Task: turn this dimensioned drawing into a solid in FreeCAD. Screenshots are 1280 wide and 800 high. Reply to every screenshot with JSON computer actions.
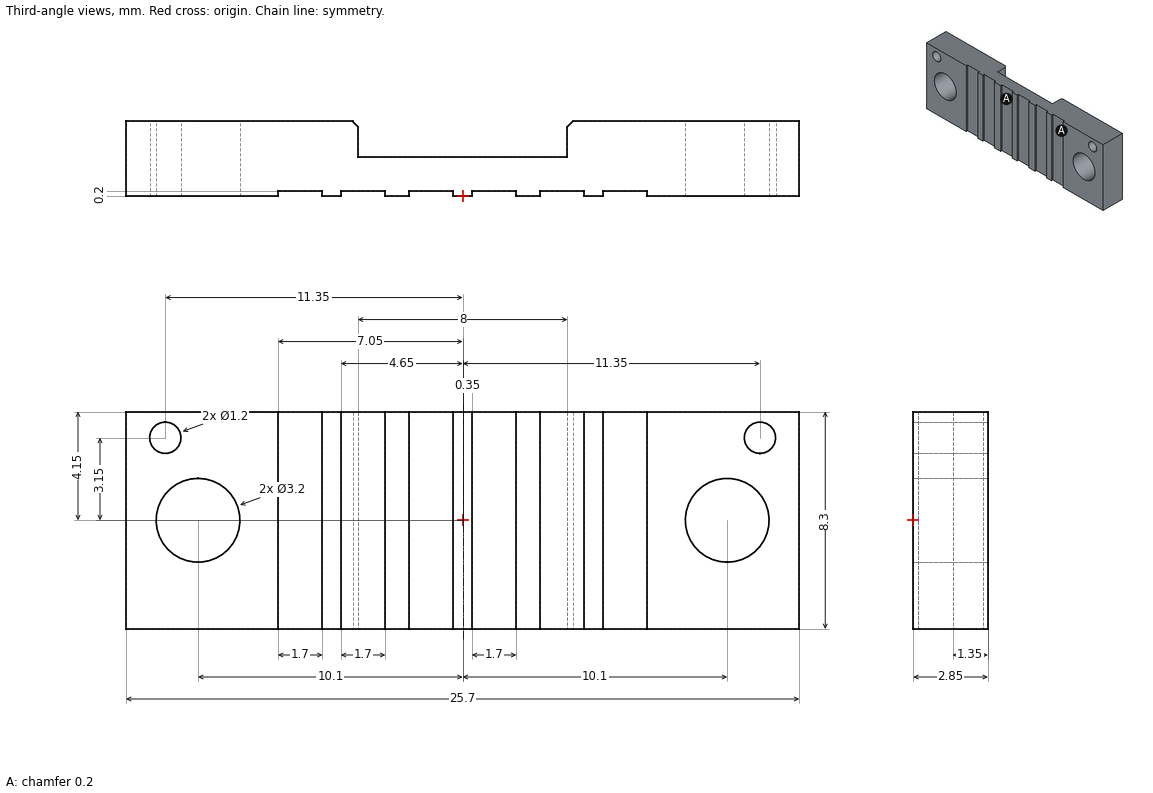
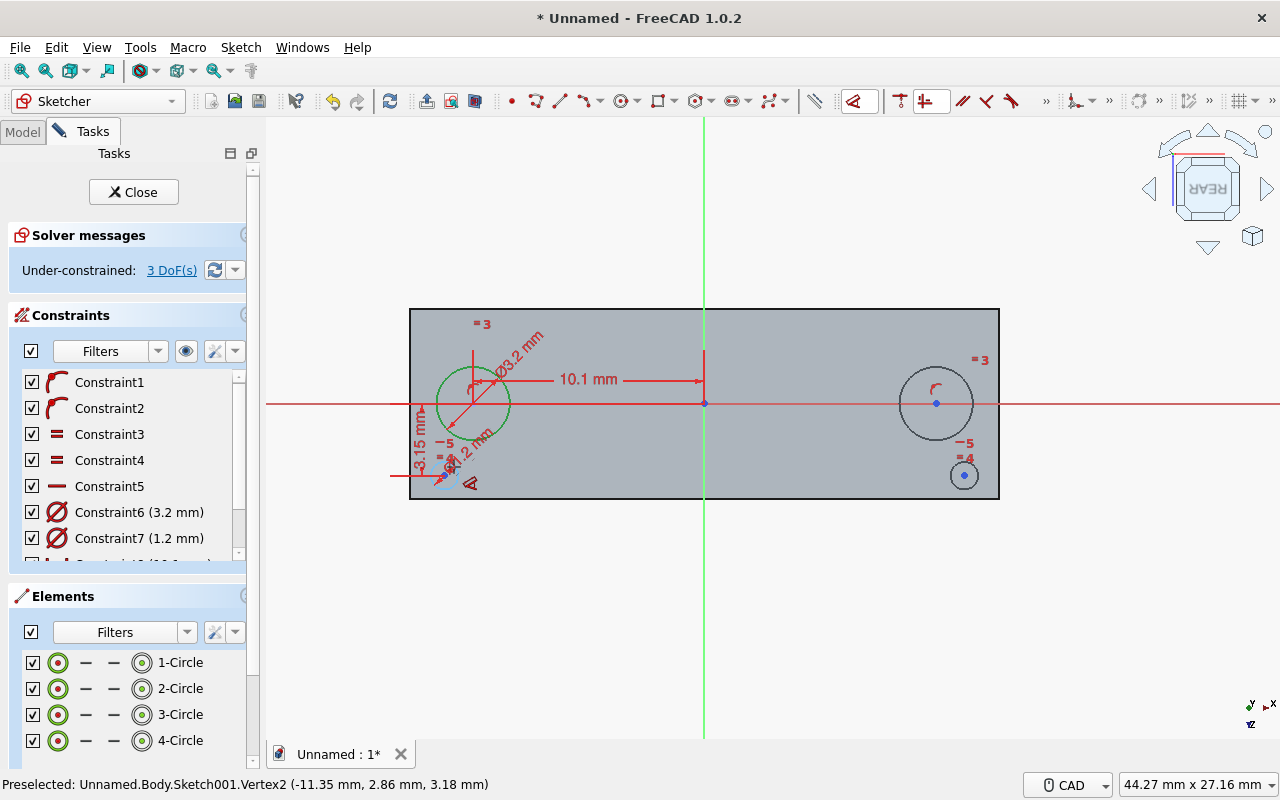
{"action": "left_click", "coordinate": [936, 404]}
{"action": "left_click", "coordinate": [820, 370]}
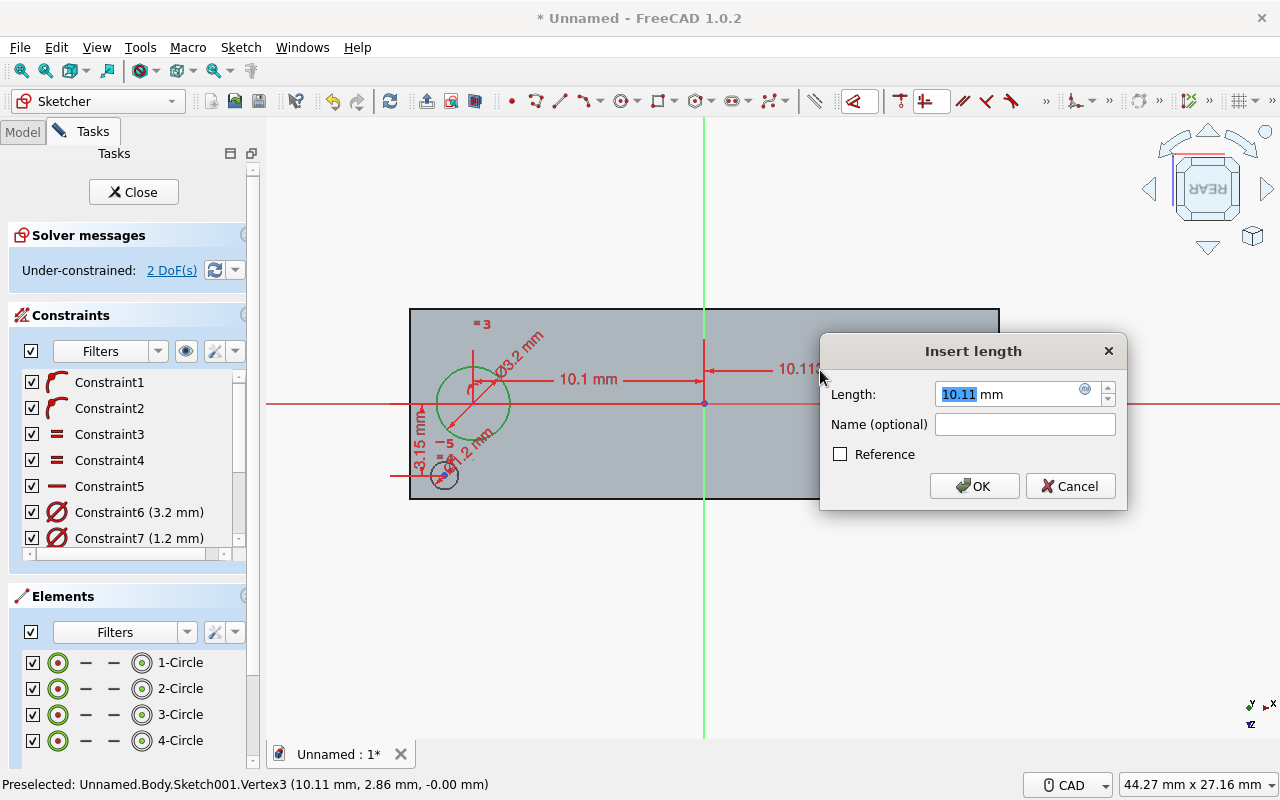
{"action": "type", "text": "10.1"}
{"action": "key", "text": "Return"}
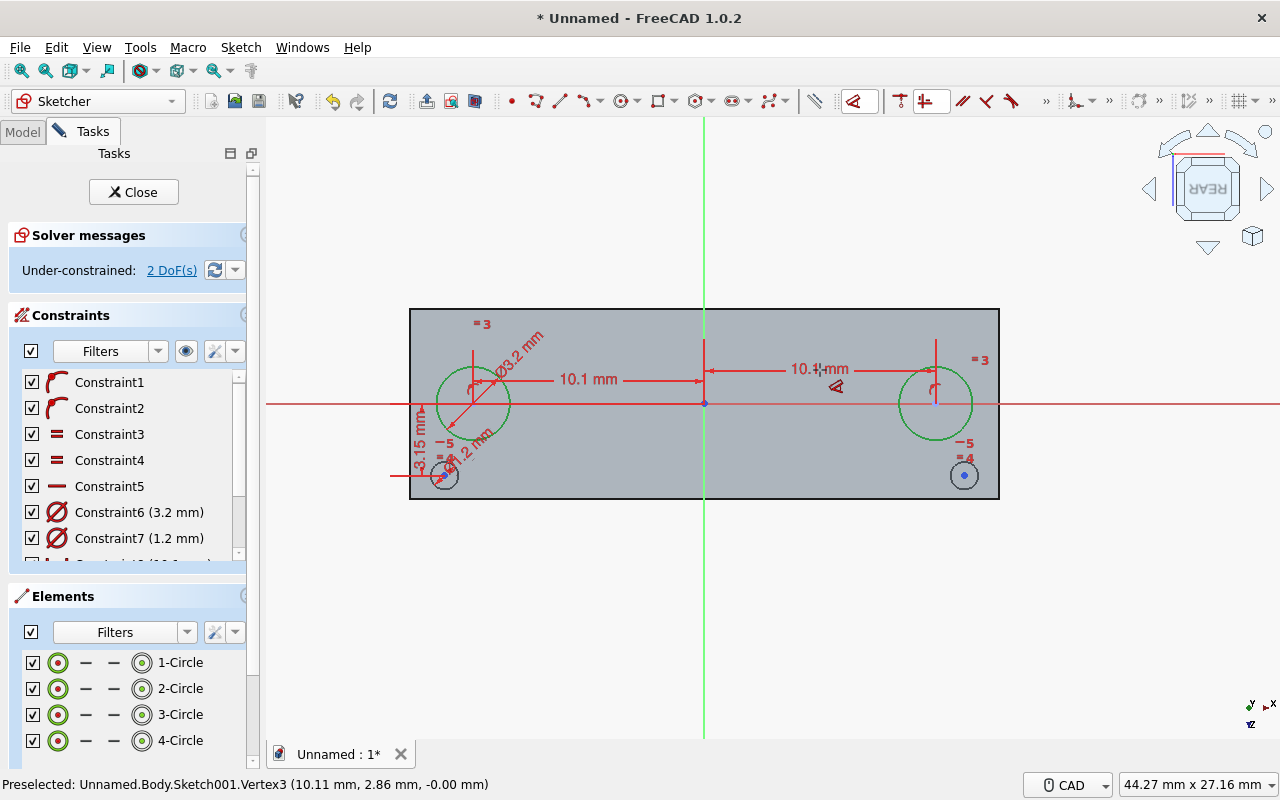
{"action": "left_click", "coordinate": [445, 476]}
{"action": "left_click", "coordinate": [575, 510]}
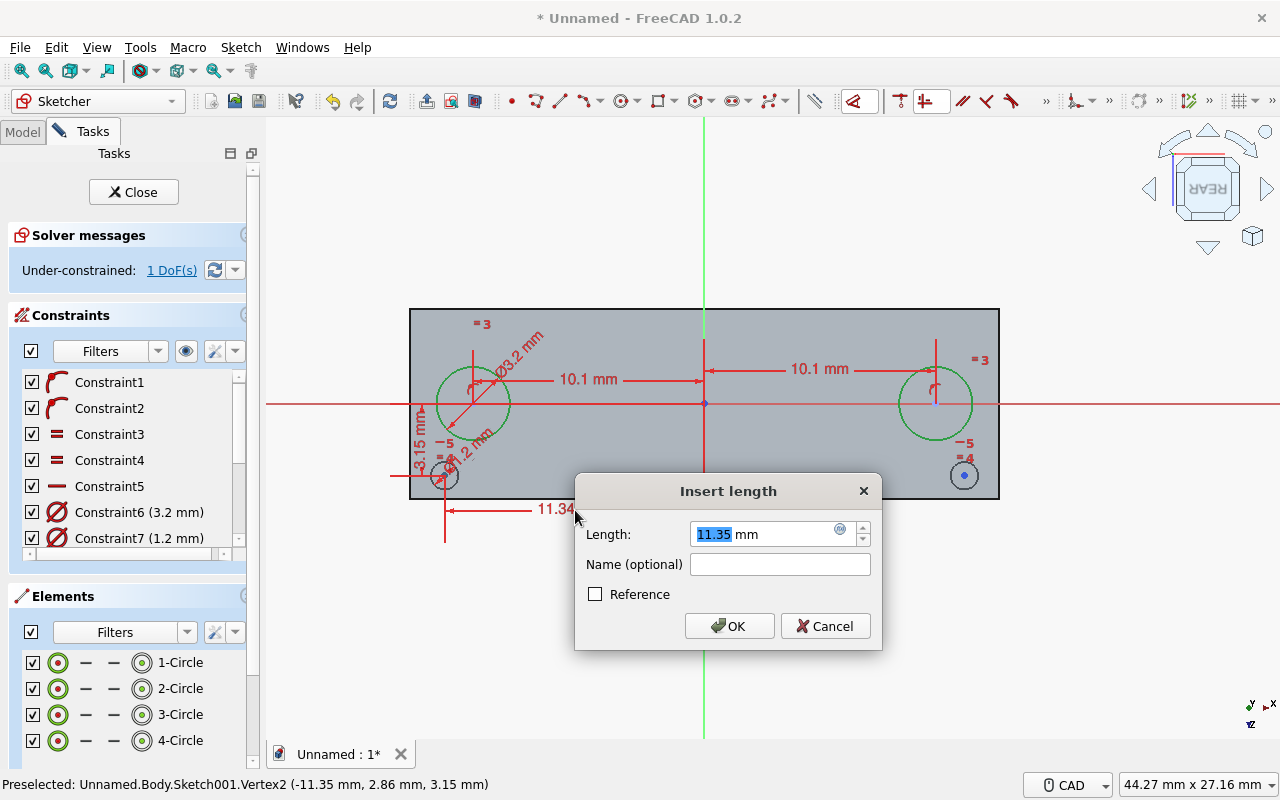
{"action": "type", "text": "11.35"}
{"action": "key", "text": "Return"}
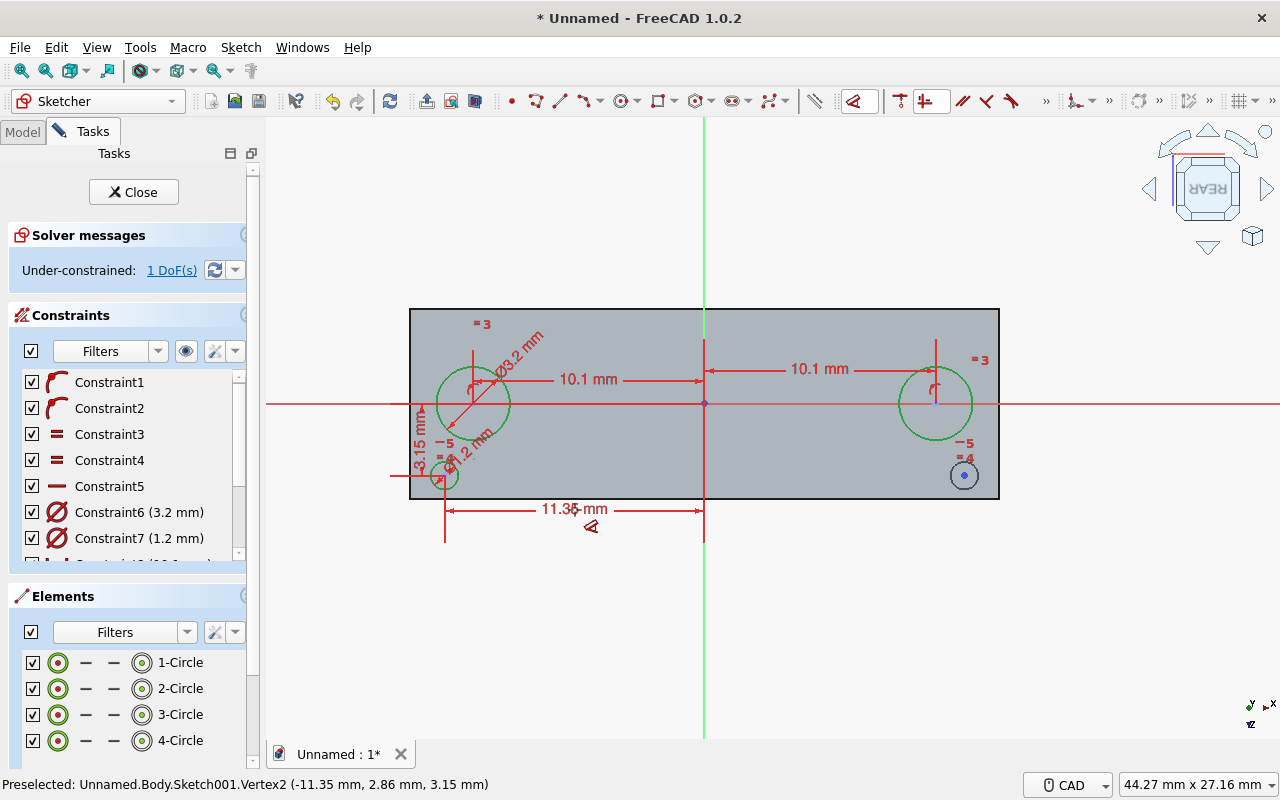
{"action": "left_click", "coordinate": [964, 476]}
{"action": "left_click", "coordinate": [834, 510]}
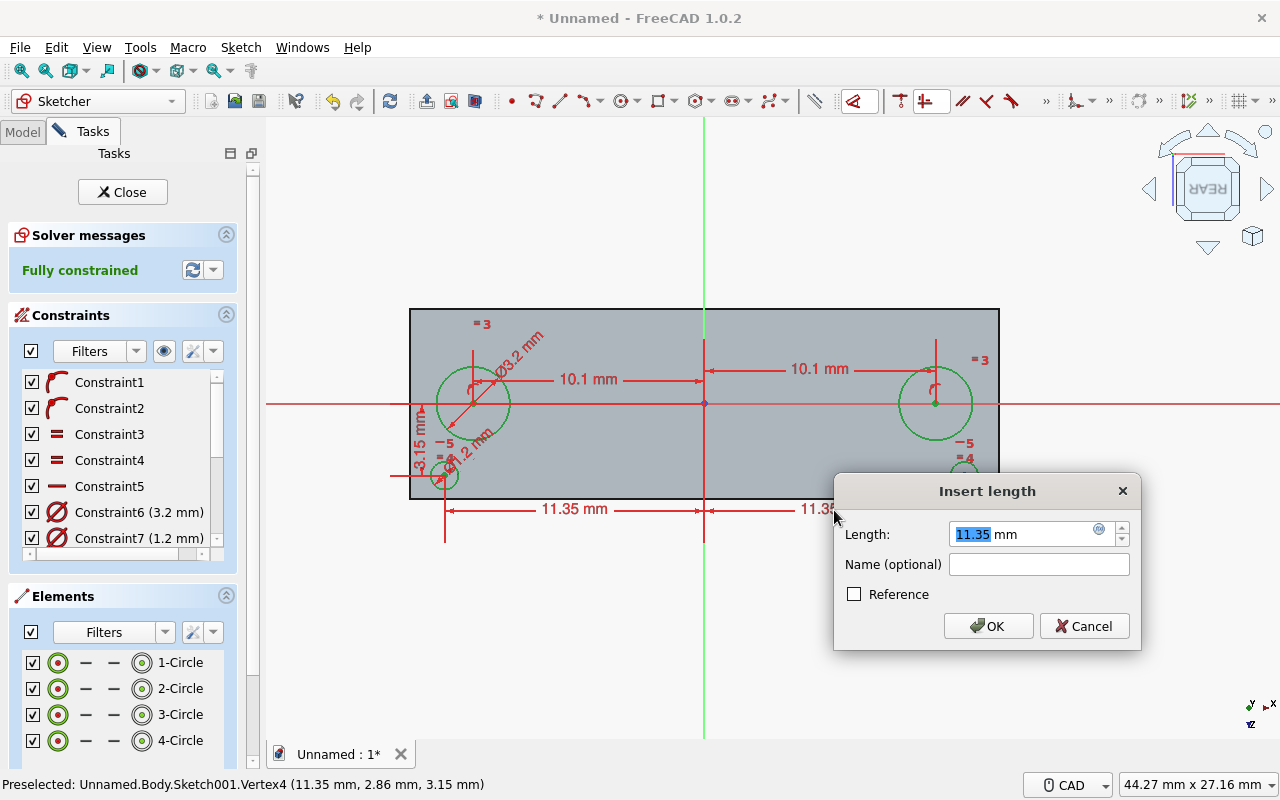
{"action": "type", "text": "11.35"}
{"action": "key", "text": "Return"}
{"action": "key", "text": "Escape"}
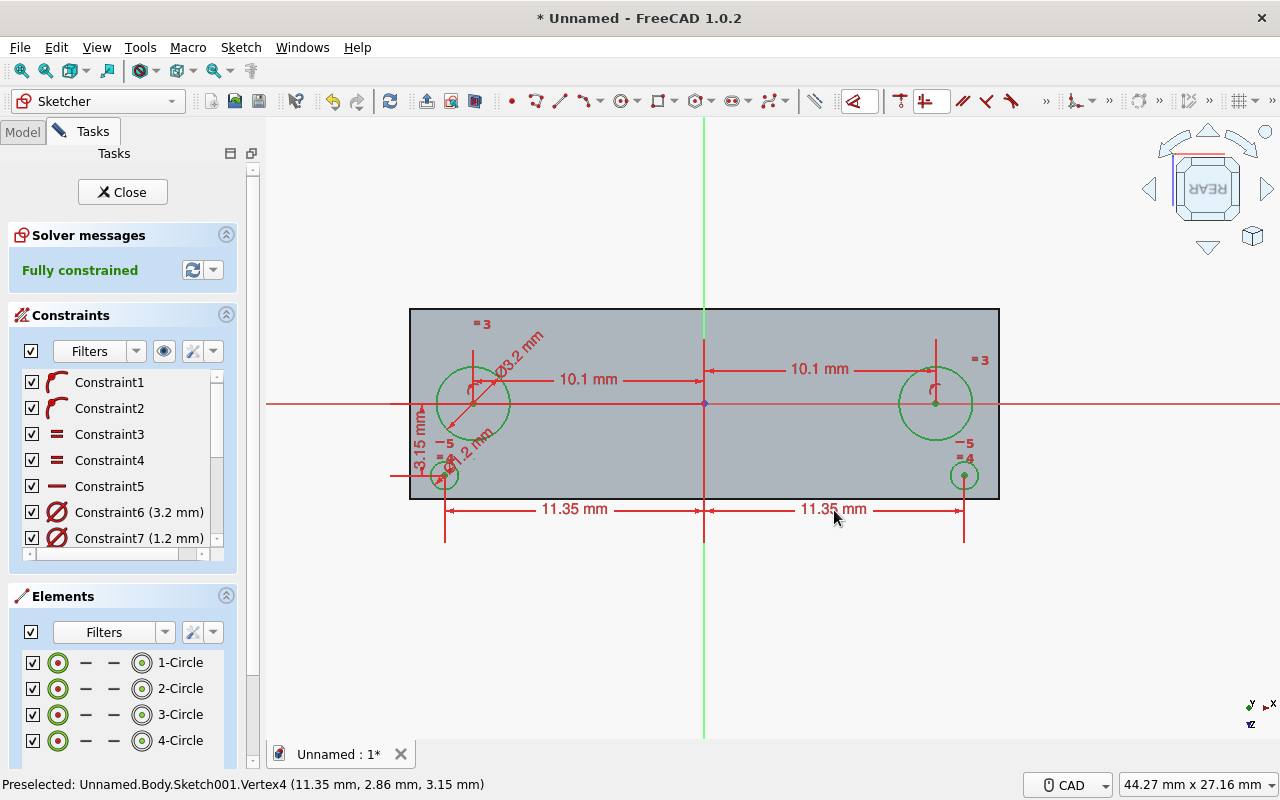
{"action": "left_click", "coordinate": [123, 192]}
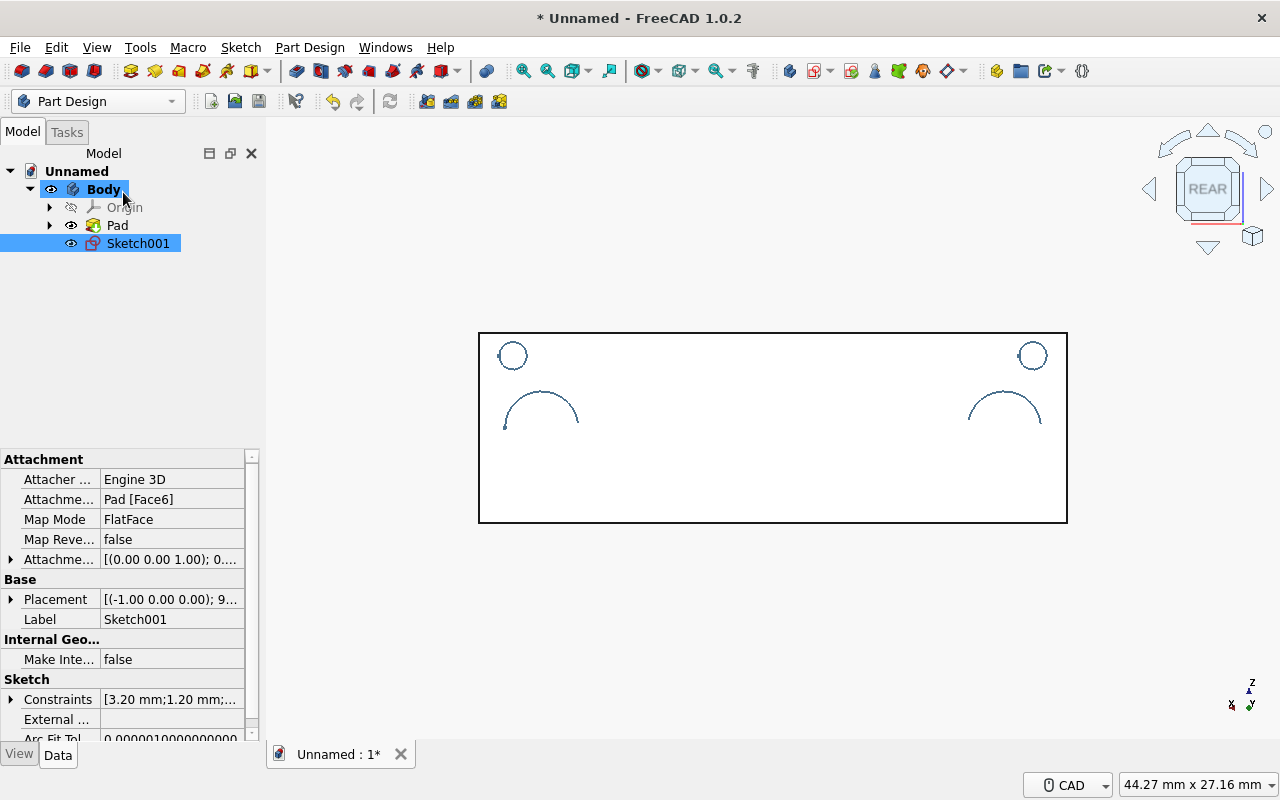
{"action": "left_click", "coordinate": [298, 72]}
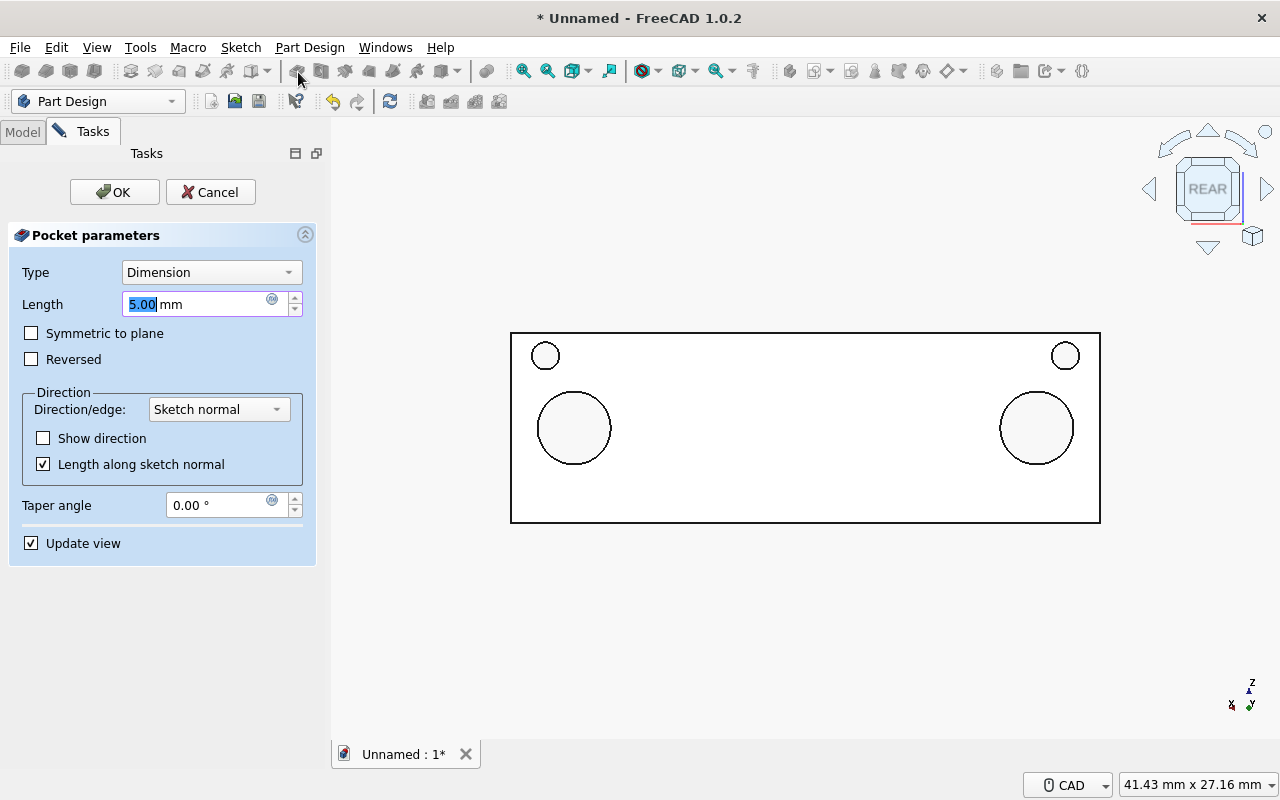
{"action": "left_click", "coordinate": [212, 272]}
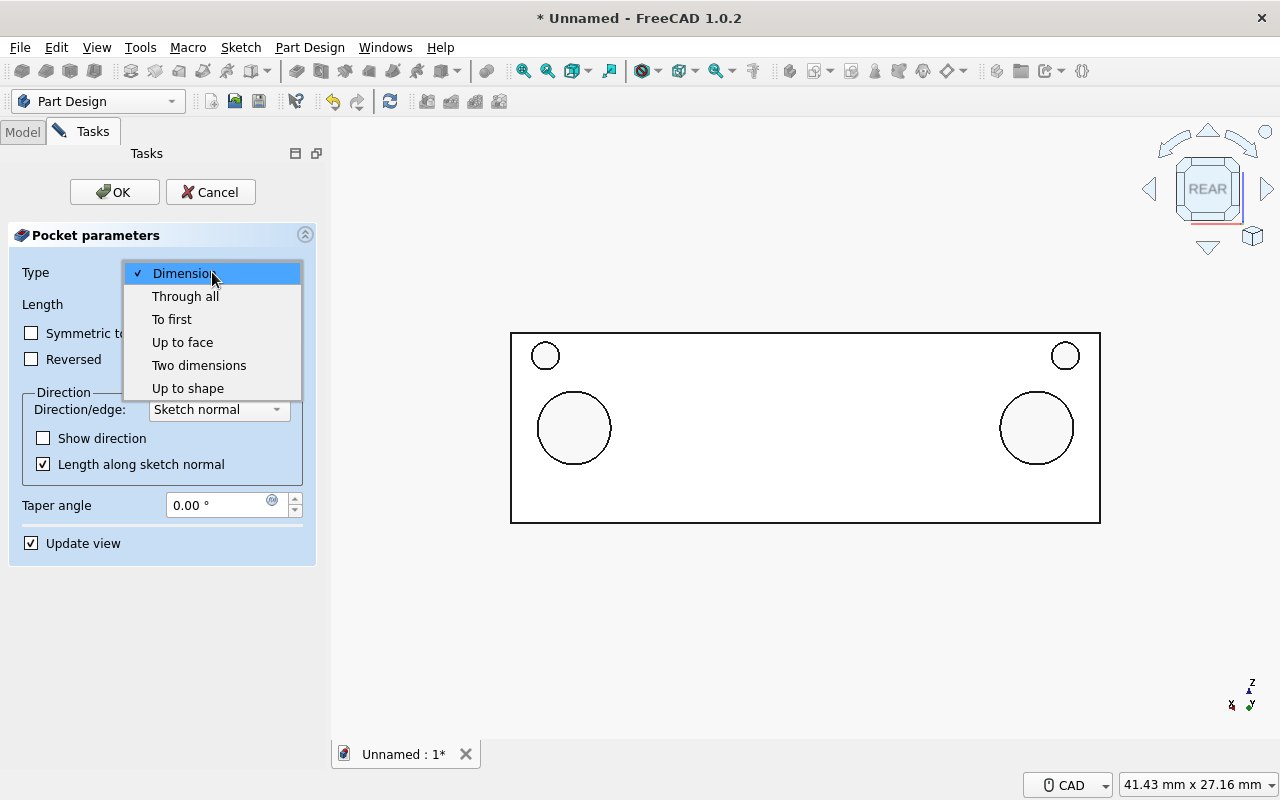
{"action": "left_click", "coordinate": [212, 296]}